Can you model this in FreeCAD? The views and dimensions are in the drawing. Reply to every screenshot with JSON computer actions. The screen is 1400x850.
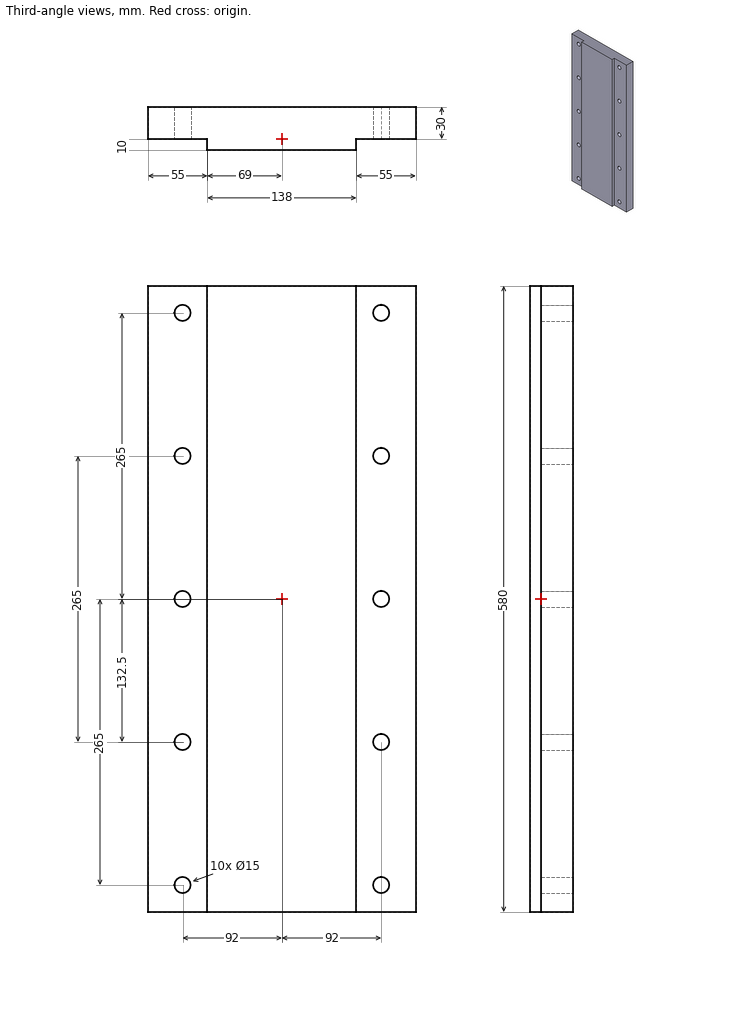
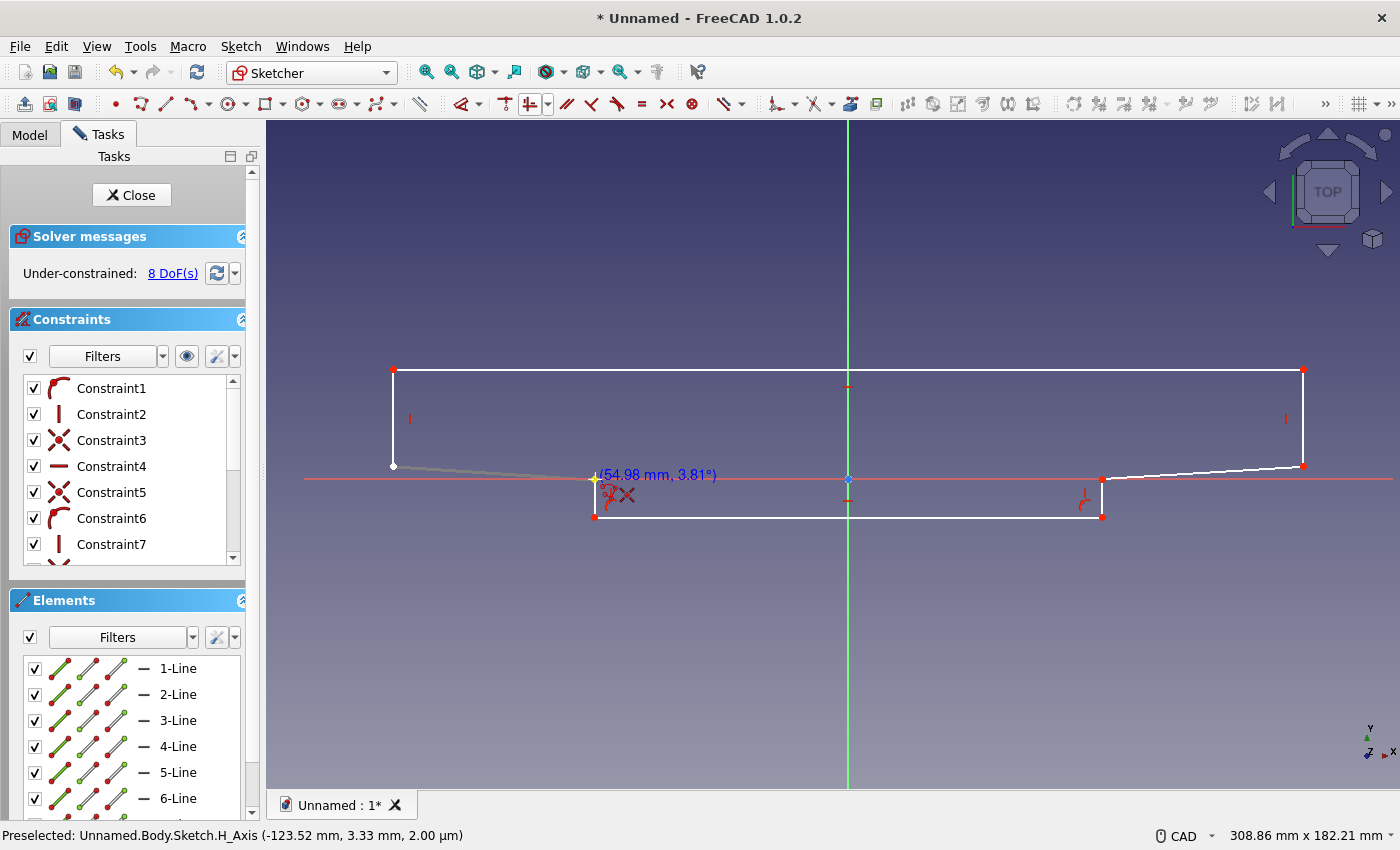
{"action": "left_click", "coordinate": [595, 479]}
{"action": "key", "text": "Escape"}
{"action": "key", "text": "Escape"}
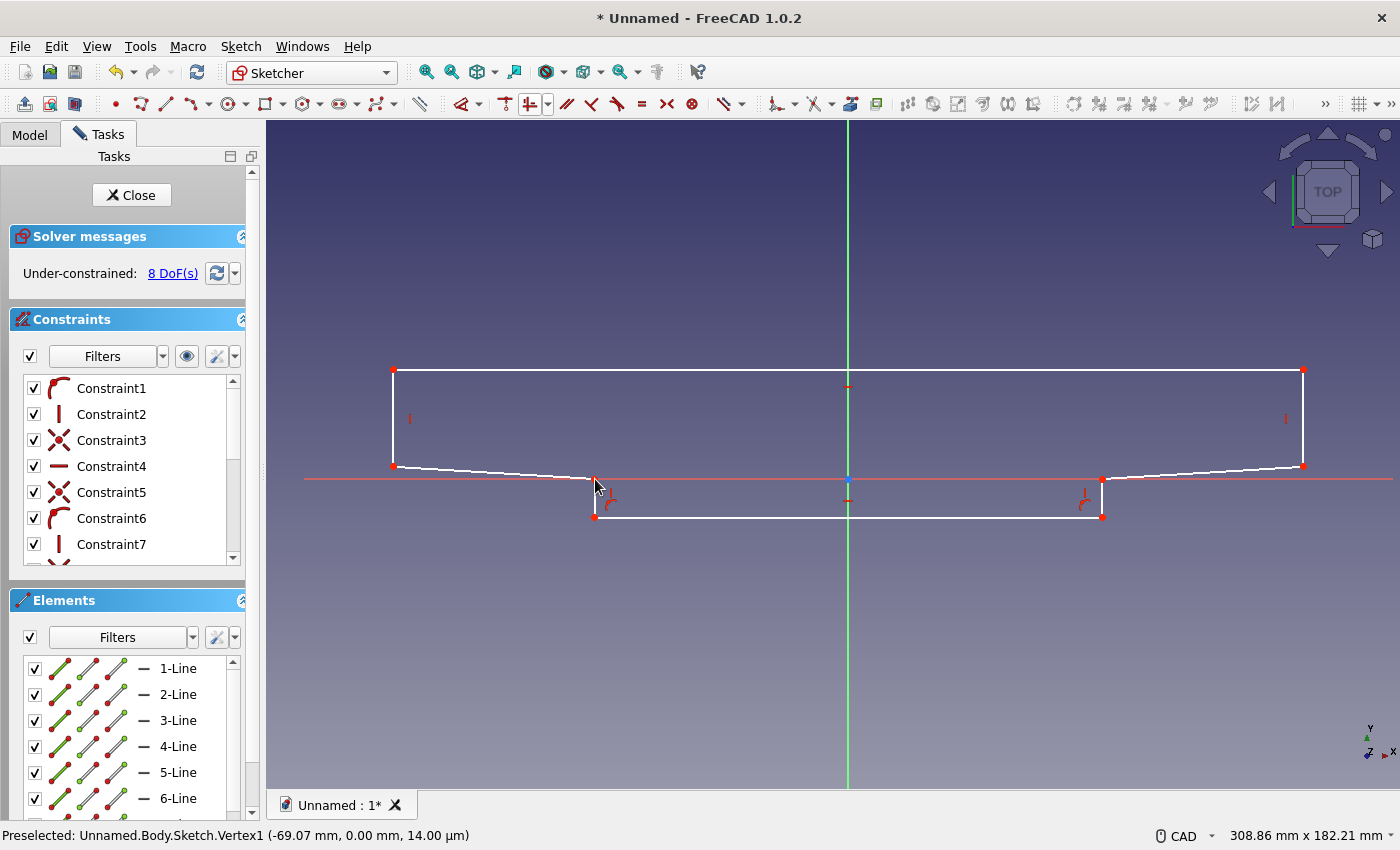
{"action": "left_click", "coordinate": [1162, 475]}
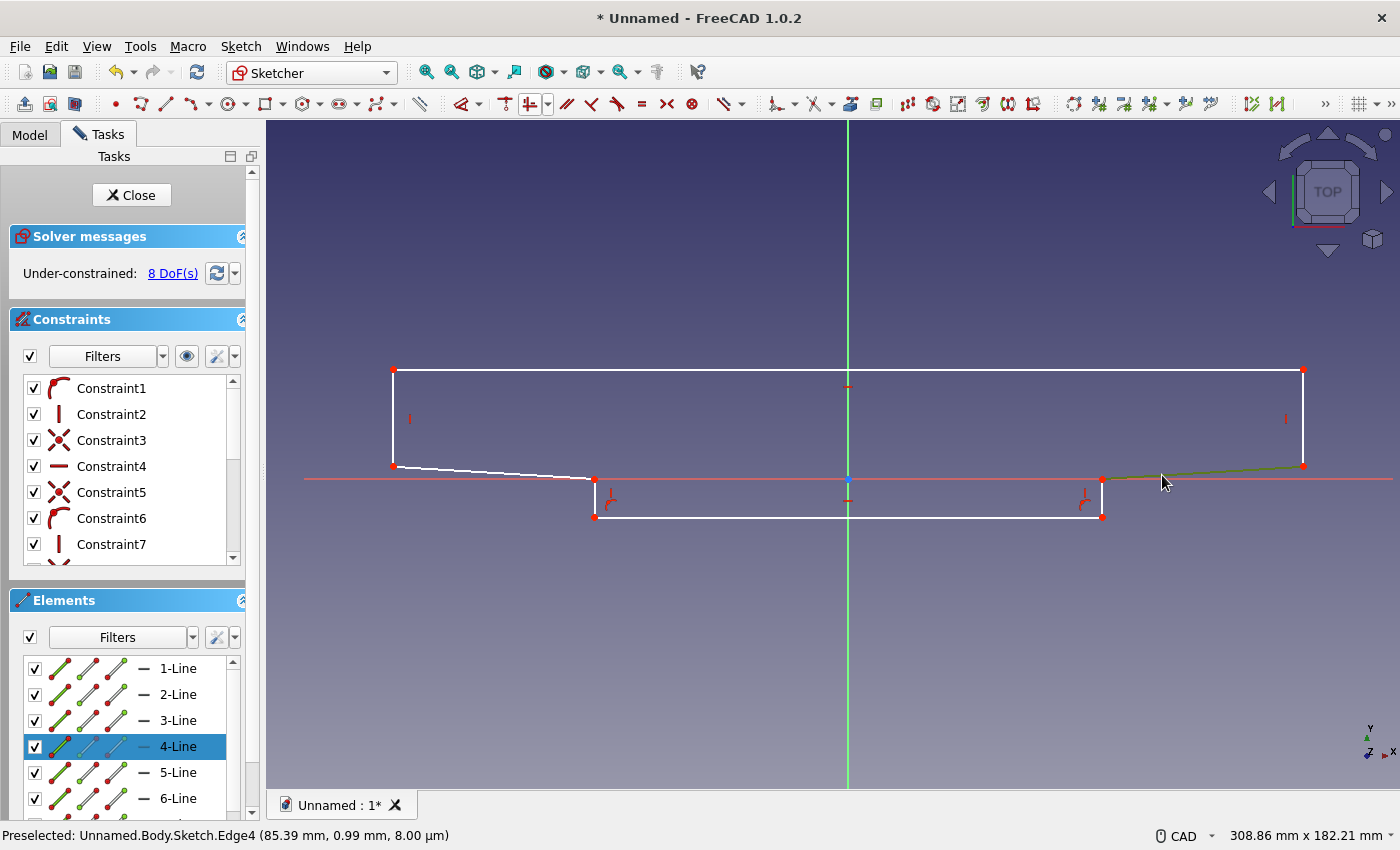
{"action": "key", "text": "h"}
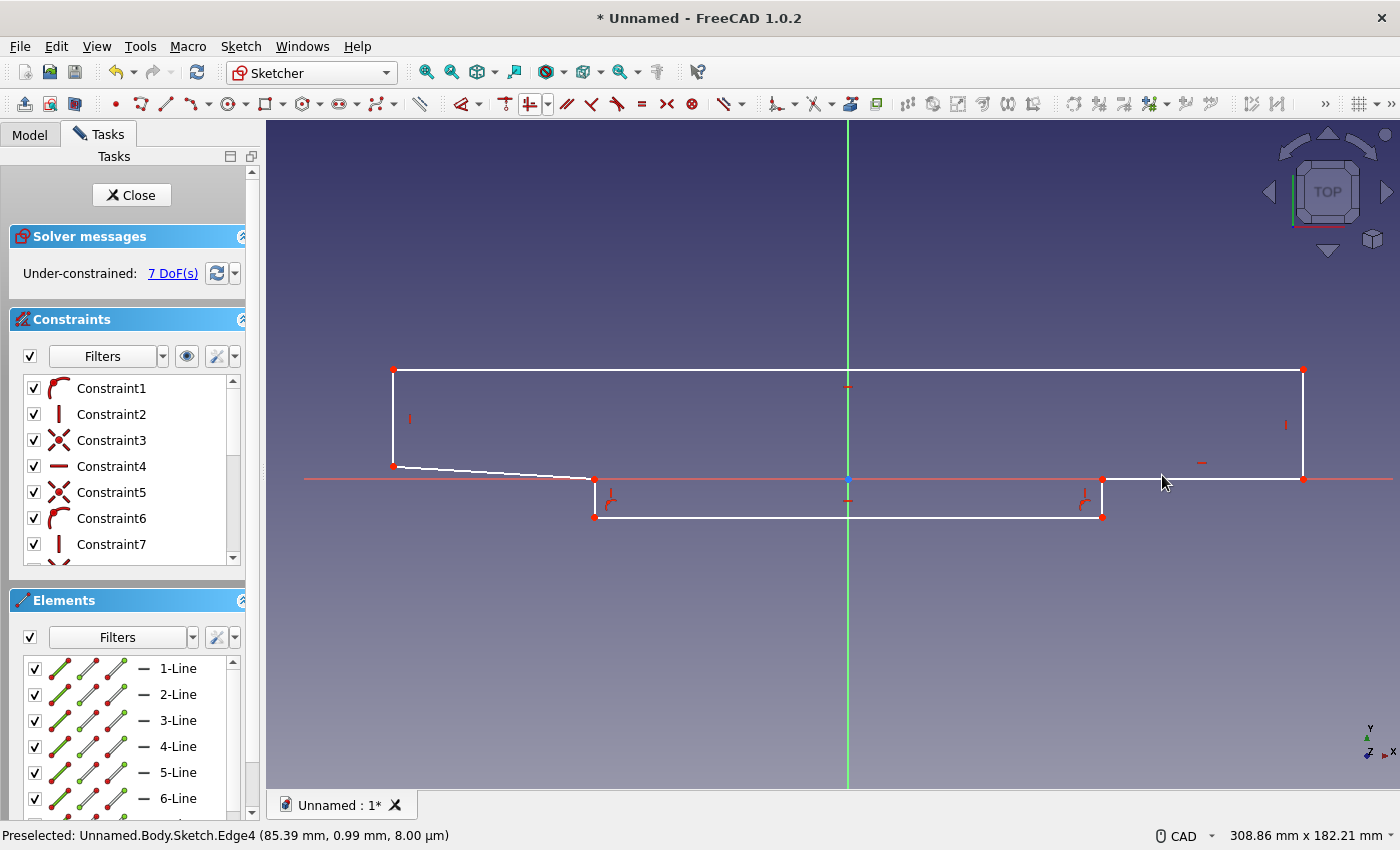
{"action": "left_click", "coordinate": [534, 475]}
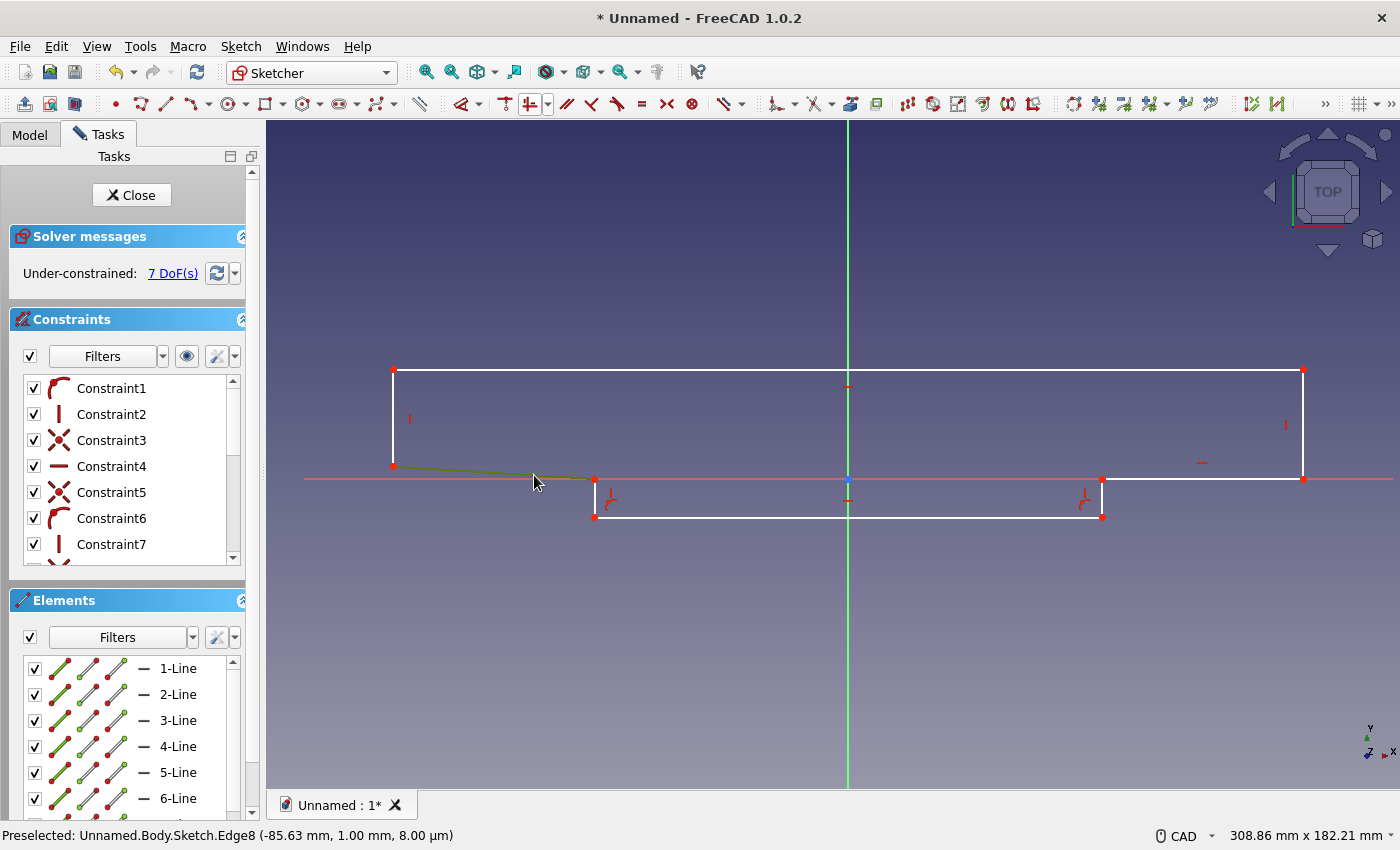
{"action": "key", "text": "h"}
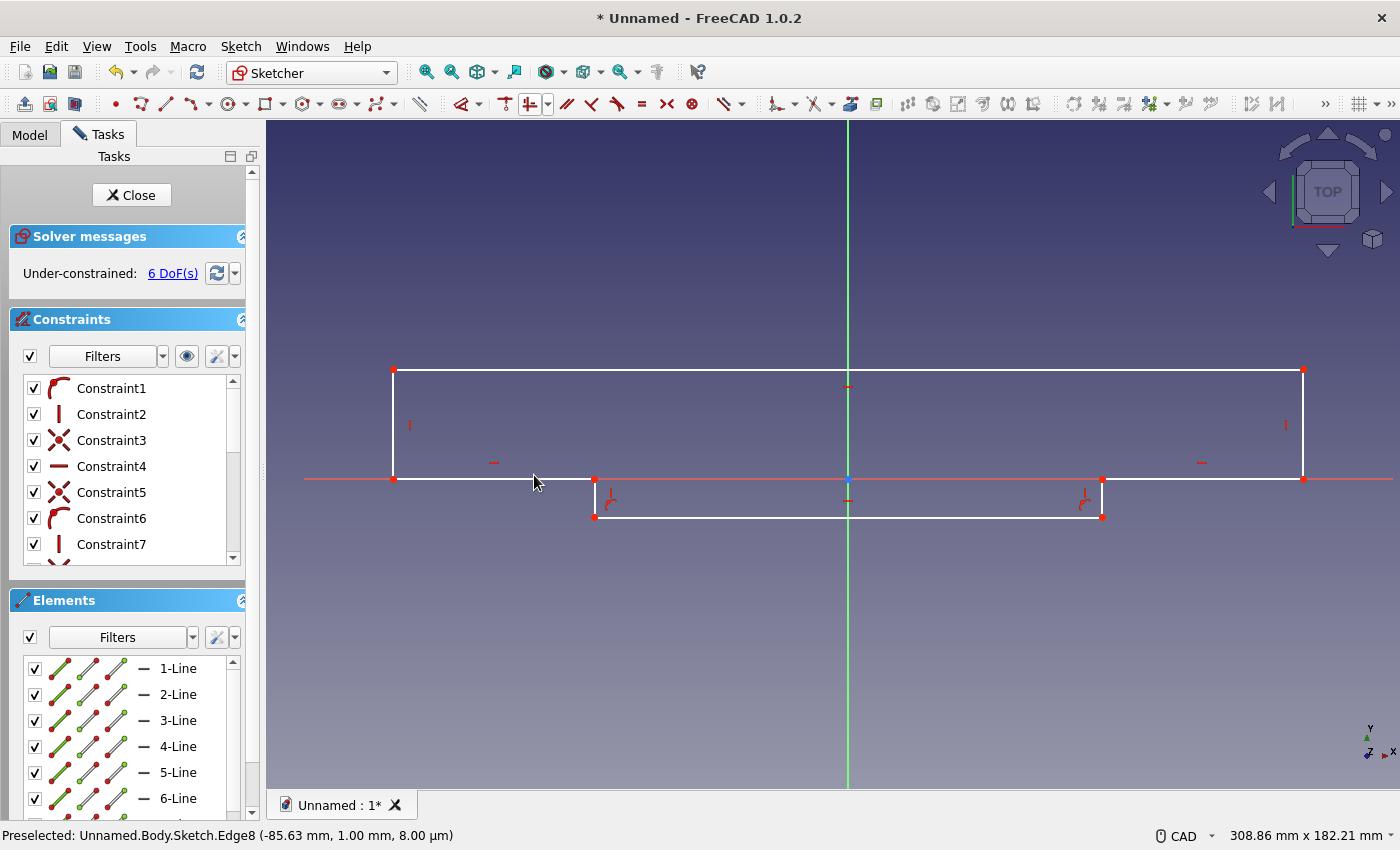
{"action": "left_click", "coordinate": [460, 104]}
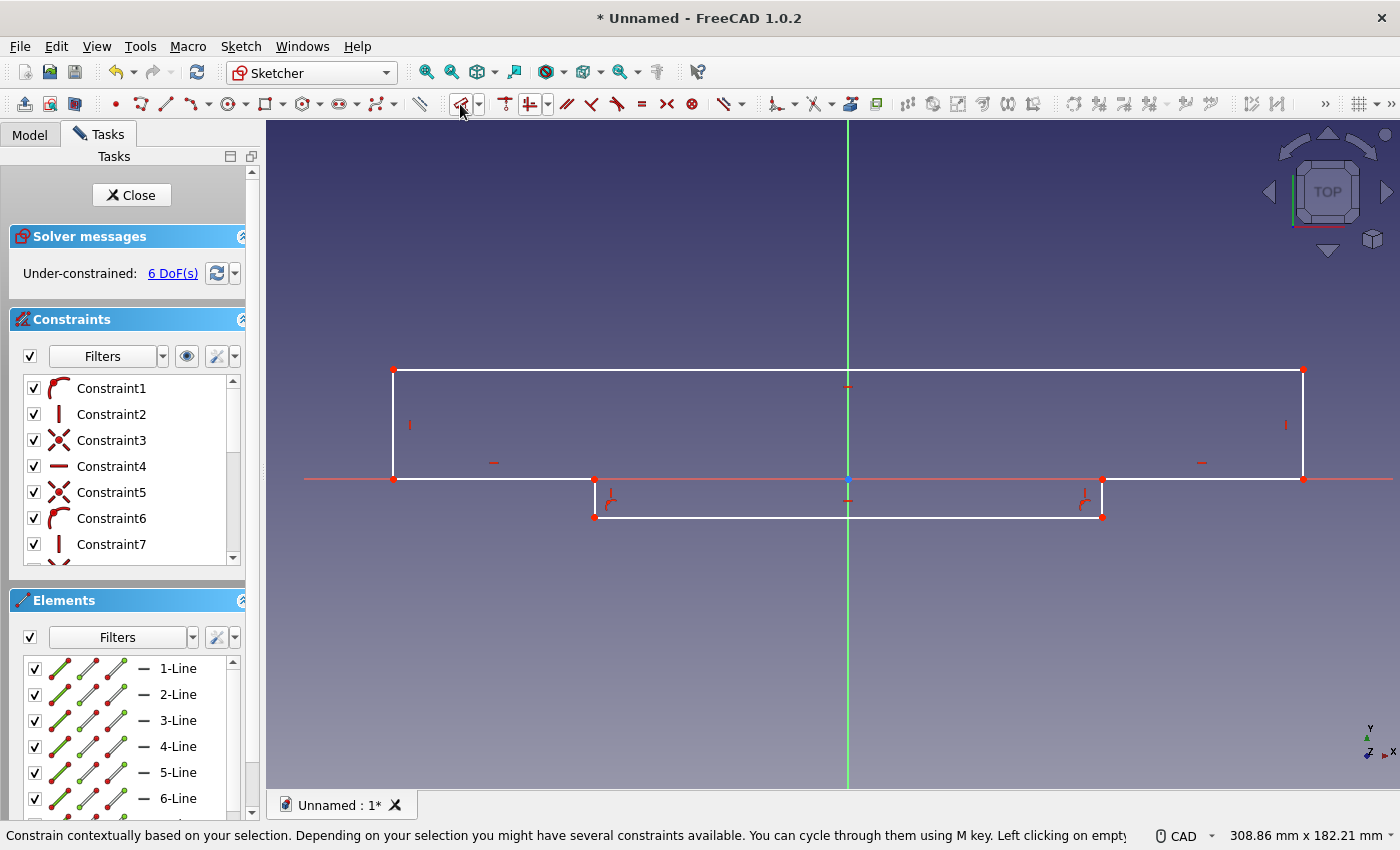
{"action": "left_click", "coordinate": [595, 491]}
{"action": "left_click", "coordinate": [561, 498]}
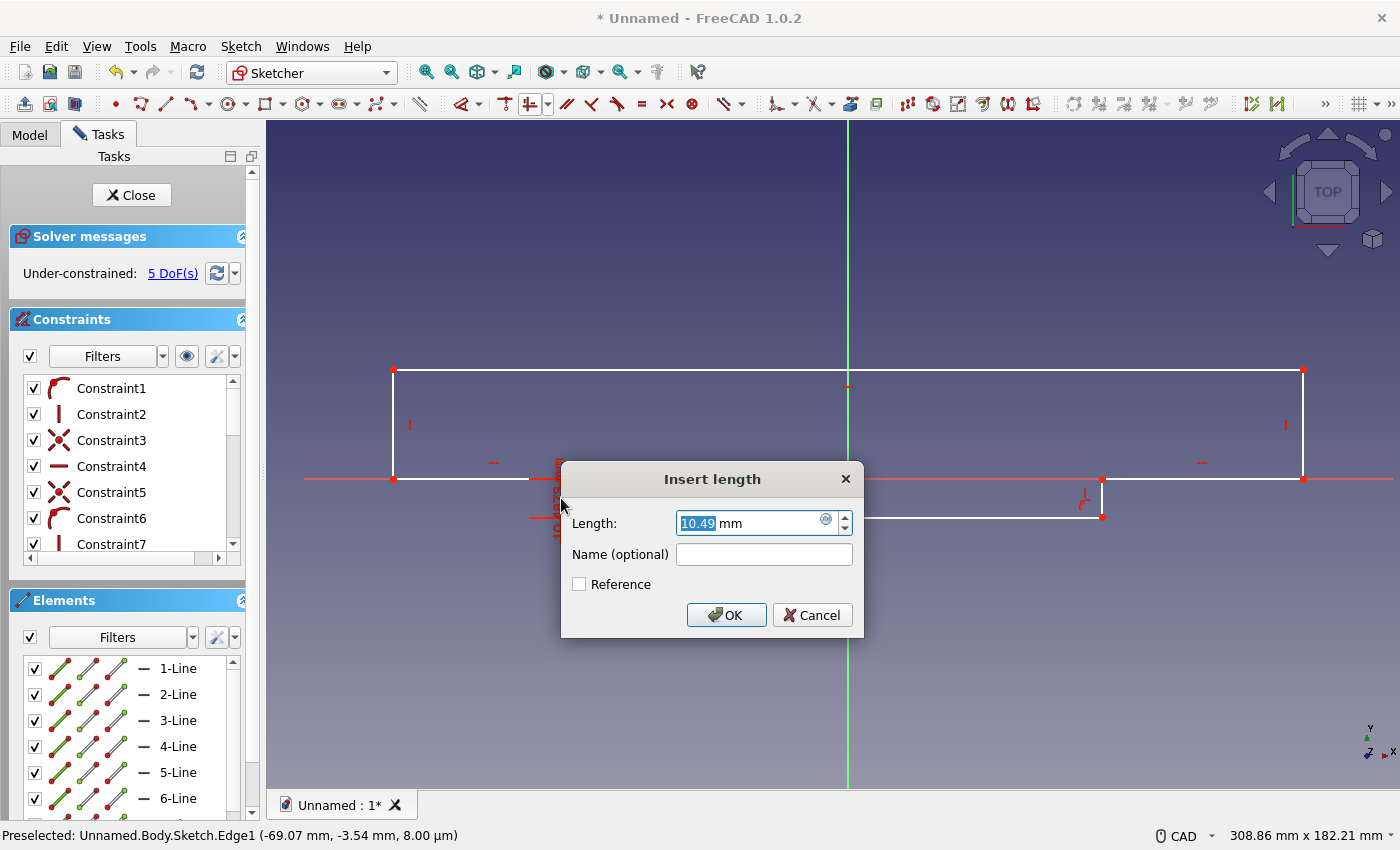
{"action": "type", "text": "10"}
{"action": "key", "text": "Return"}